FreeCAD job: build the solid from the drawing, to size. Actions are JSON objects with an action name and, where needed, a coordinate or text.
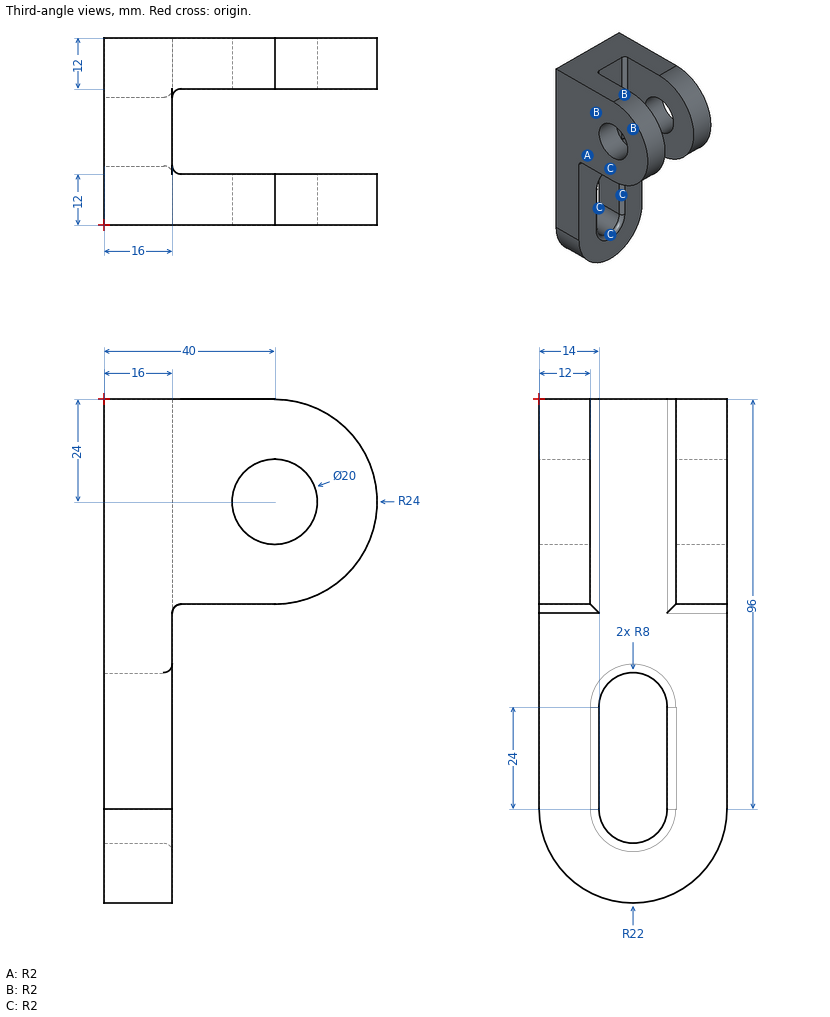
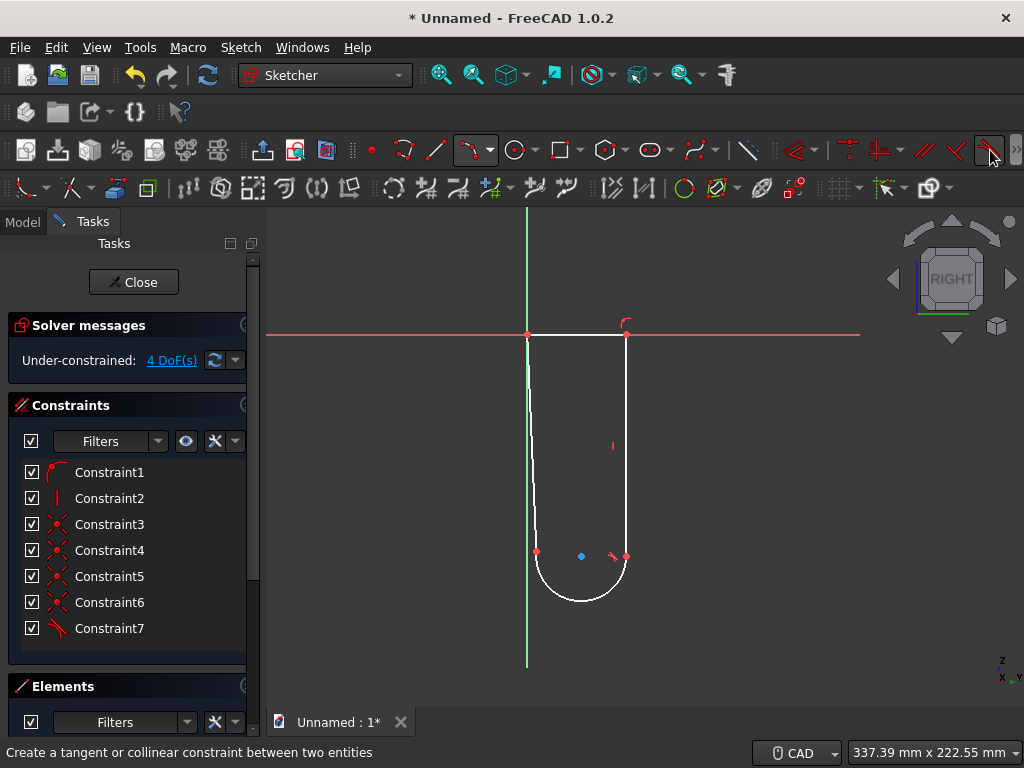
{"action": "left_click", "coordinate": [530, 400]}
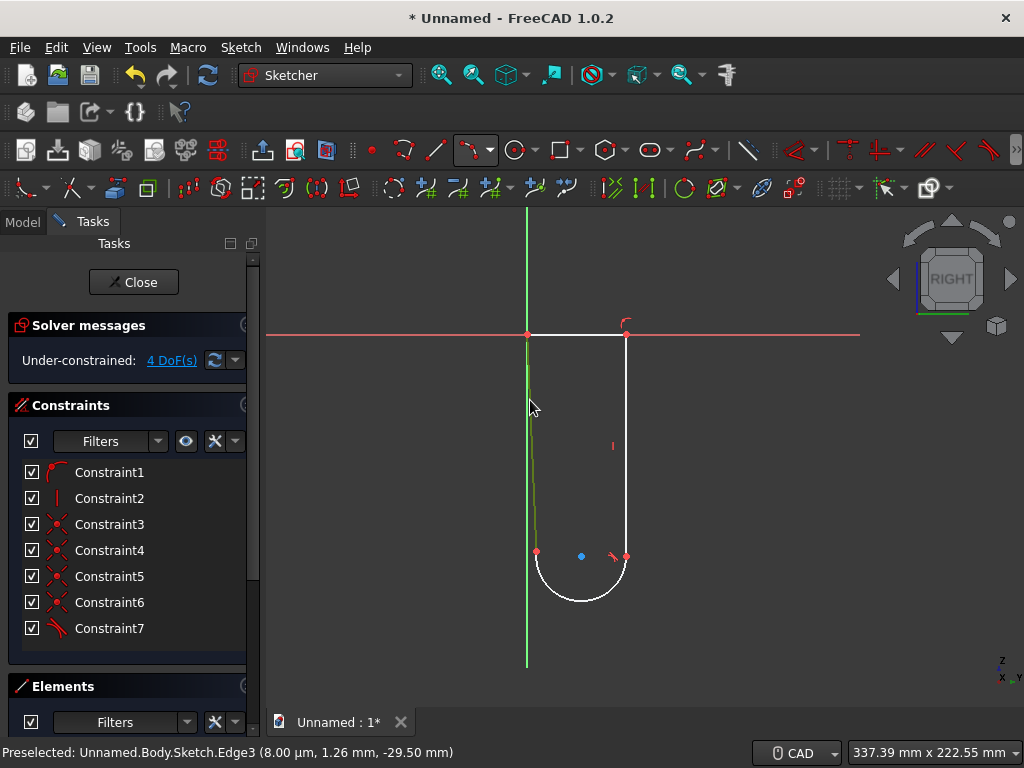
{"action": "left_click", "coordinate": [552, 591]}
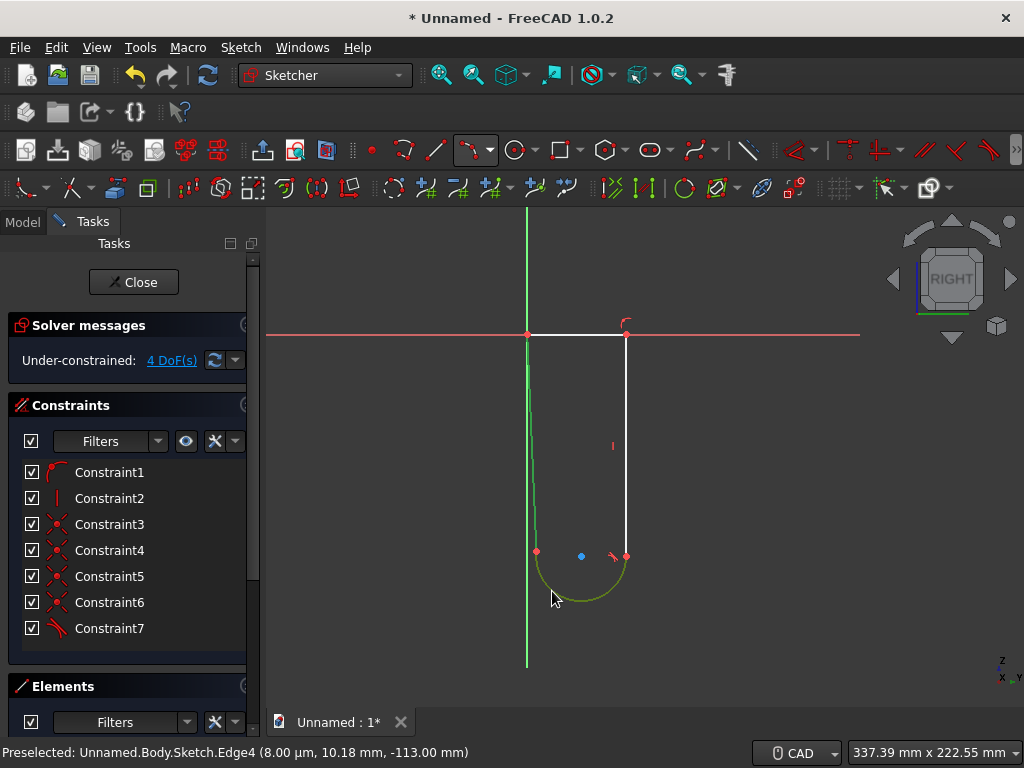
{"action": "left_click", "coordinate": [990, 150]}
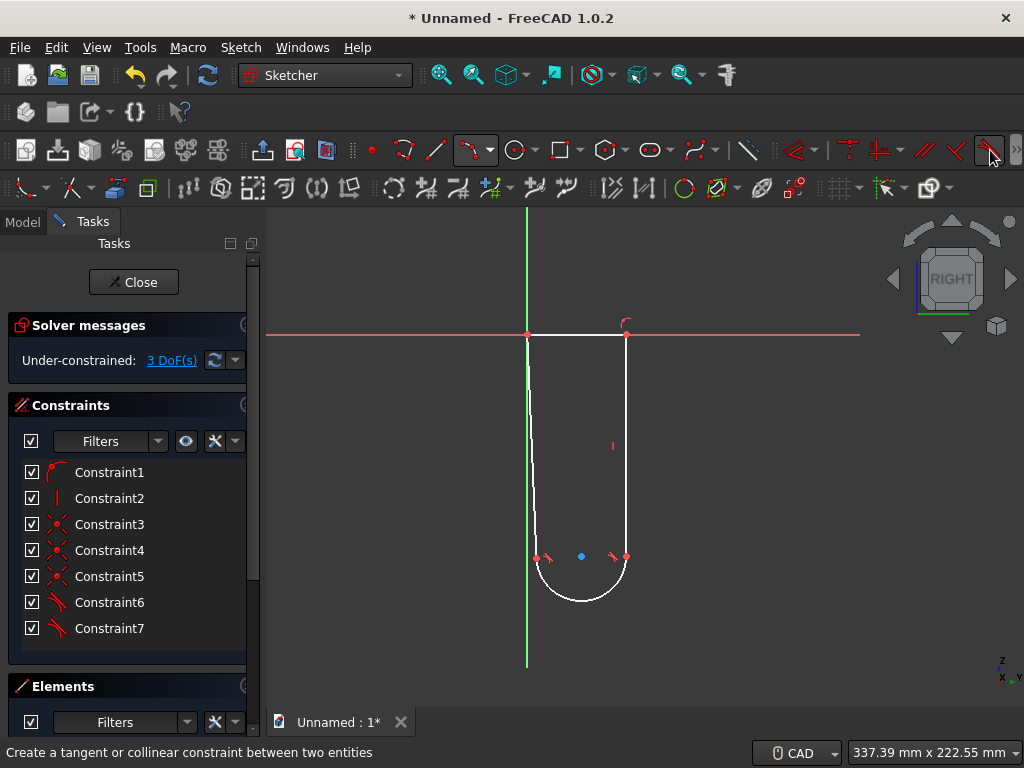
{"action": "left_click", "coordinate": [530, 402]}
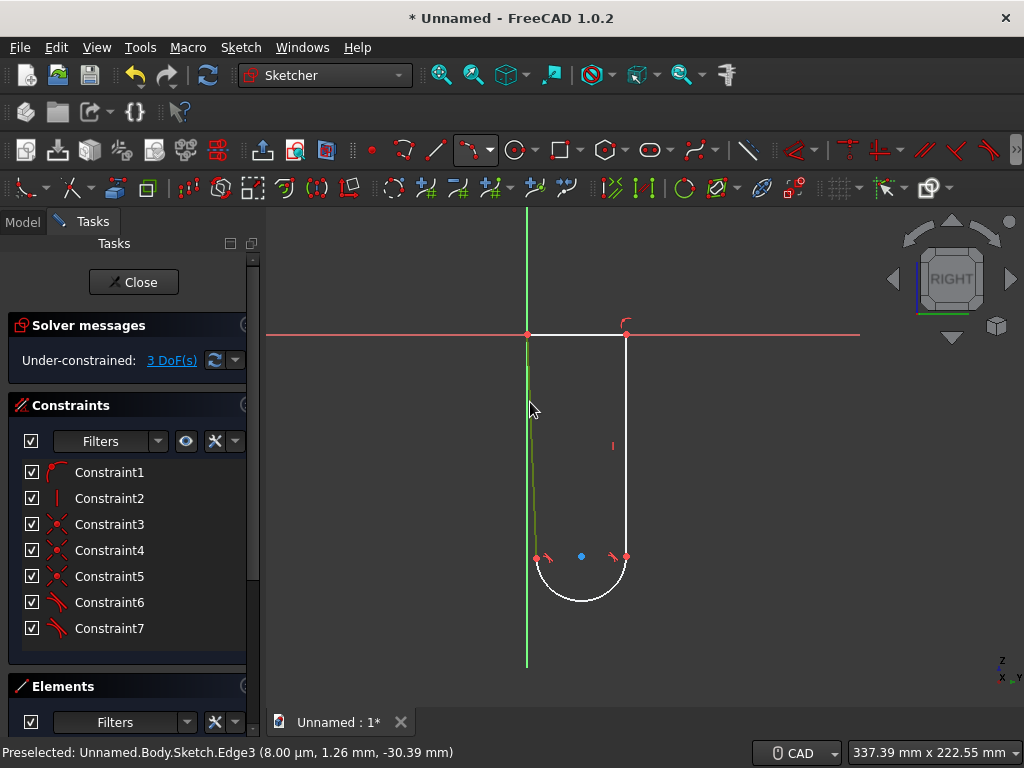
{"action": "left_click", "coordinate": [902, 150]}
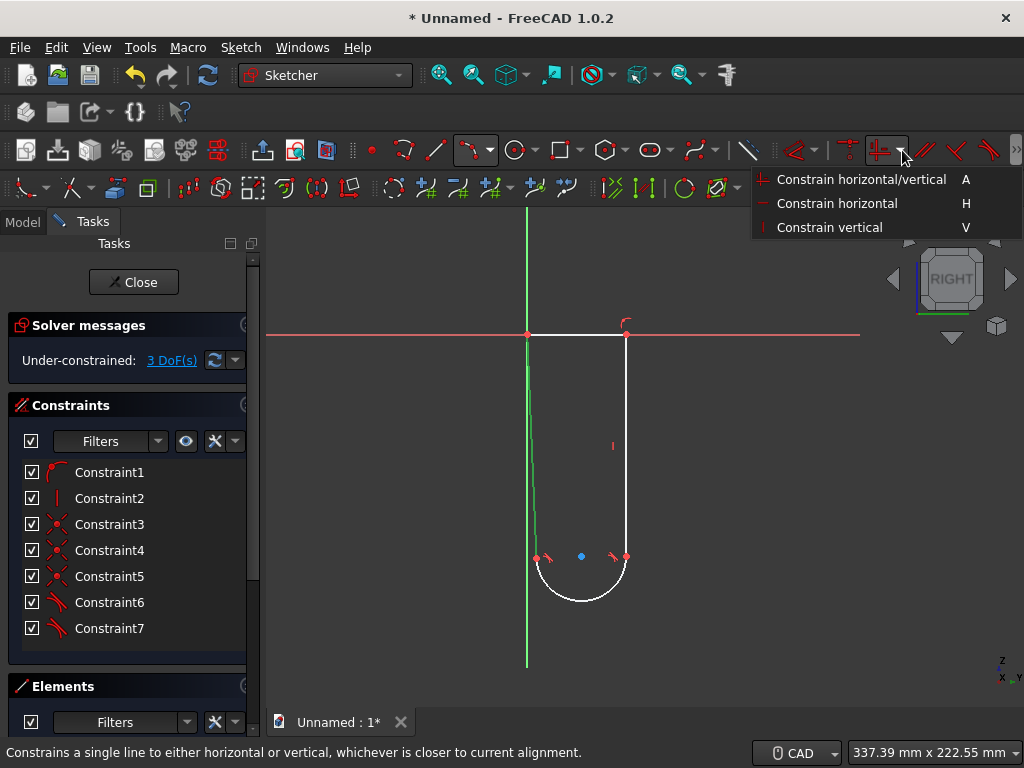
{"action": "left_click", "coordinate": [887, 227]}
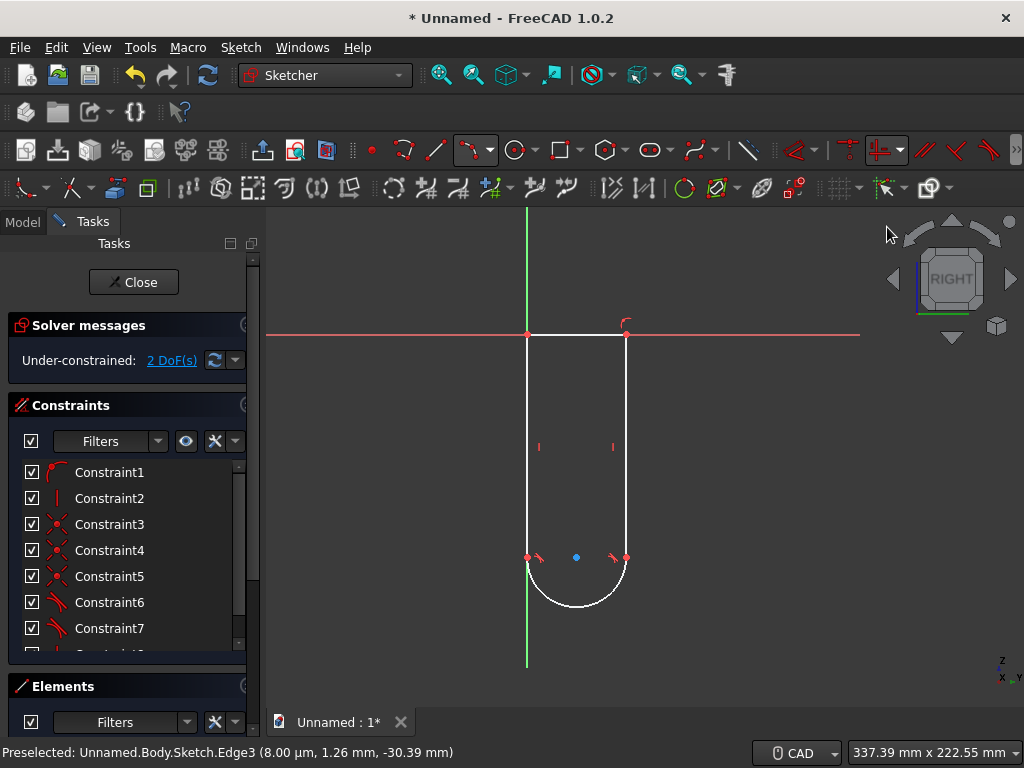
{"action": "left_click", "coordinate": [794, 150]}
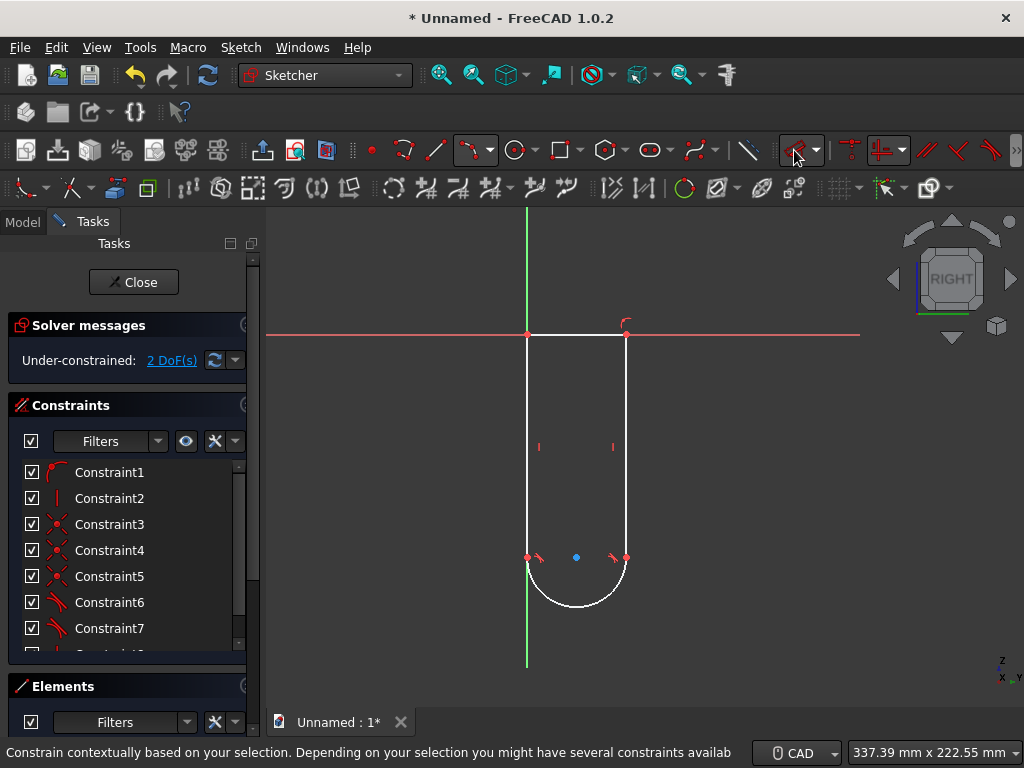
{"action": "left_click", "coordinate": [548, 598]}
{"action": "left_click", "coordinate": [503, 593]}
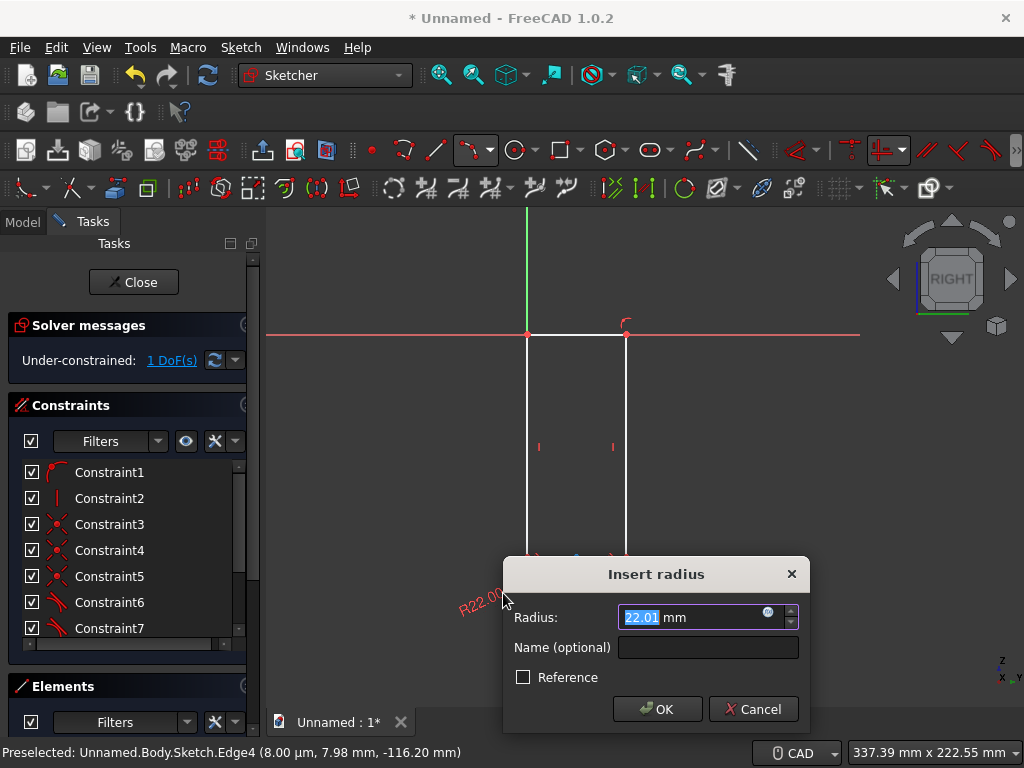
{"action": "type", "text": "22"}
{"action": "key", "text": "Return"}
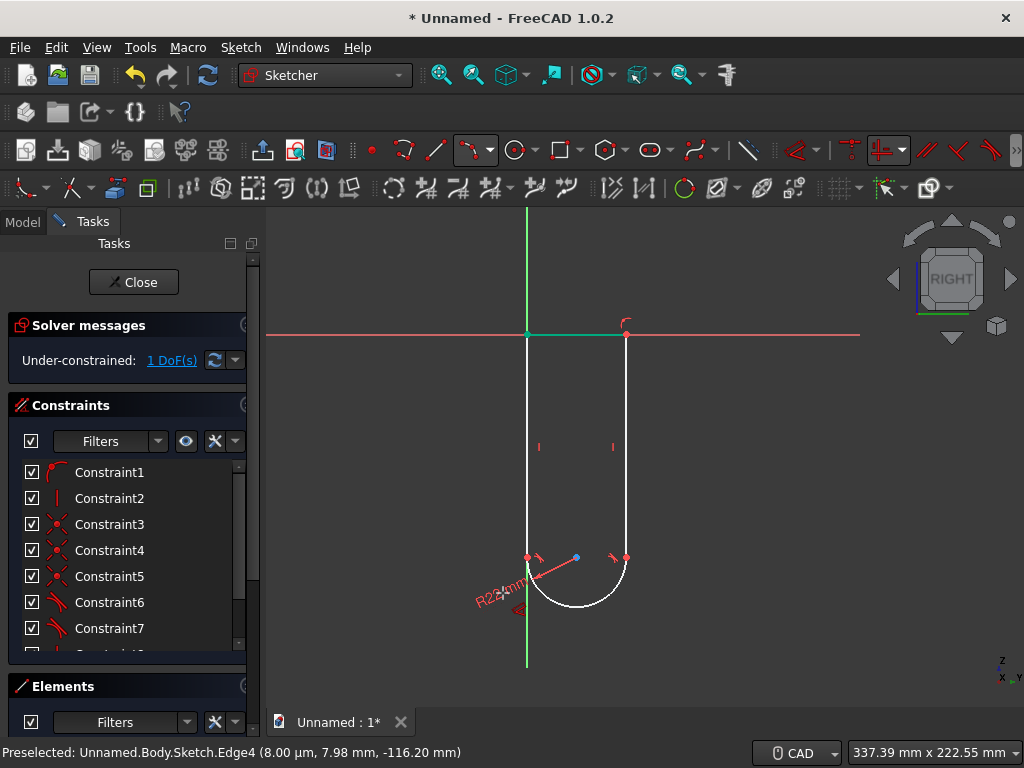
{"action": "left_click", "coordinate": [626, 491]}
{"action": "left_click", "coordinate": [660, 446]}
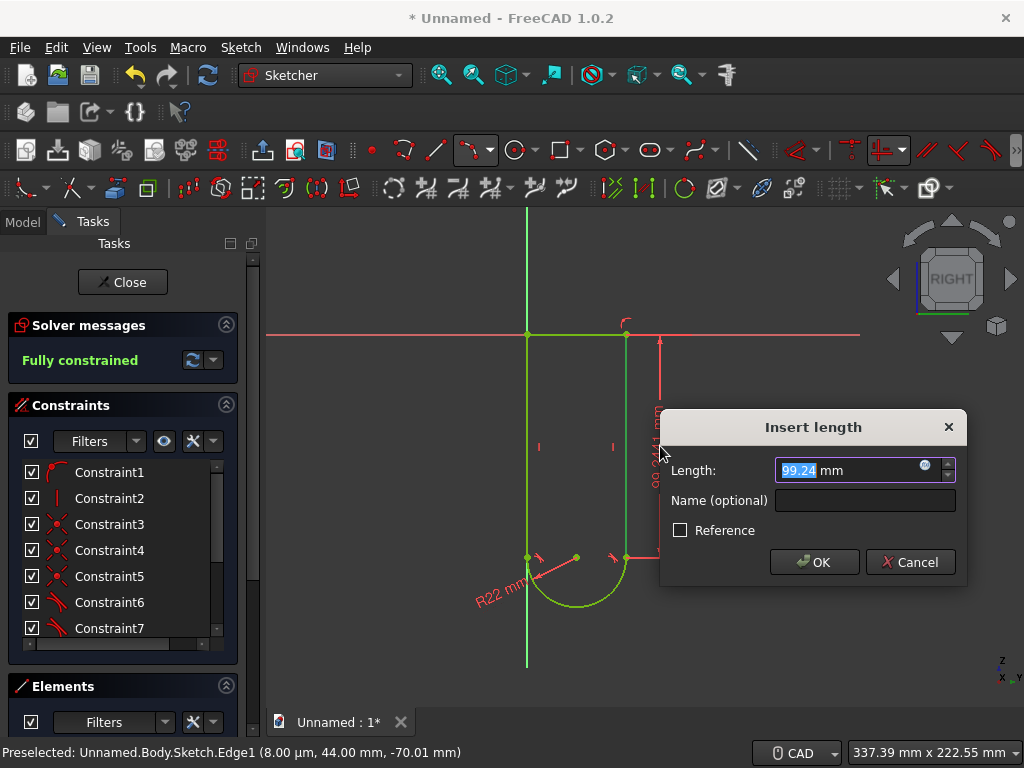
{"action": "type", "text": "96"}
{"action": "key", "text": "Return"}
{"action": "key", "text": "Escape"}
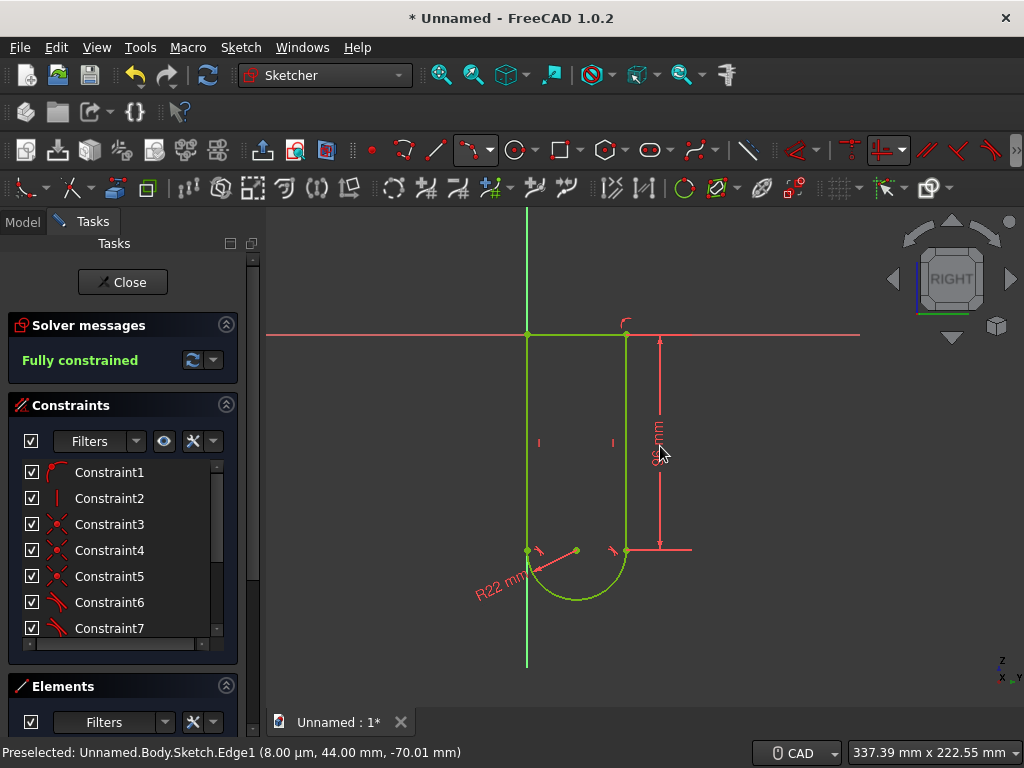
{"action": "left_click", "coordinate": [123, 282]}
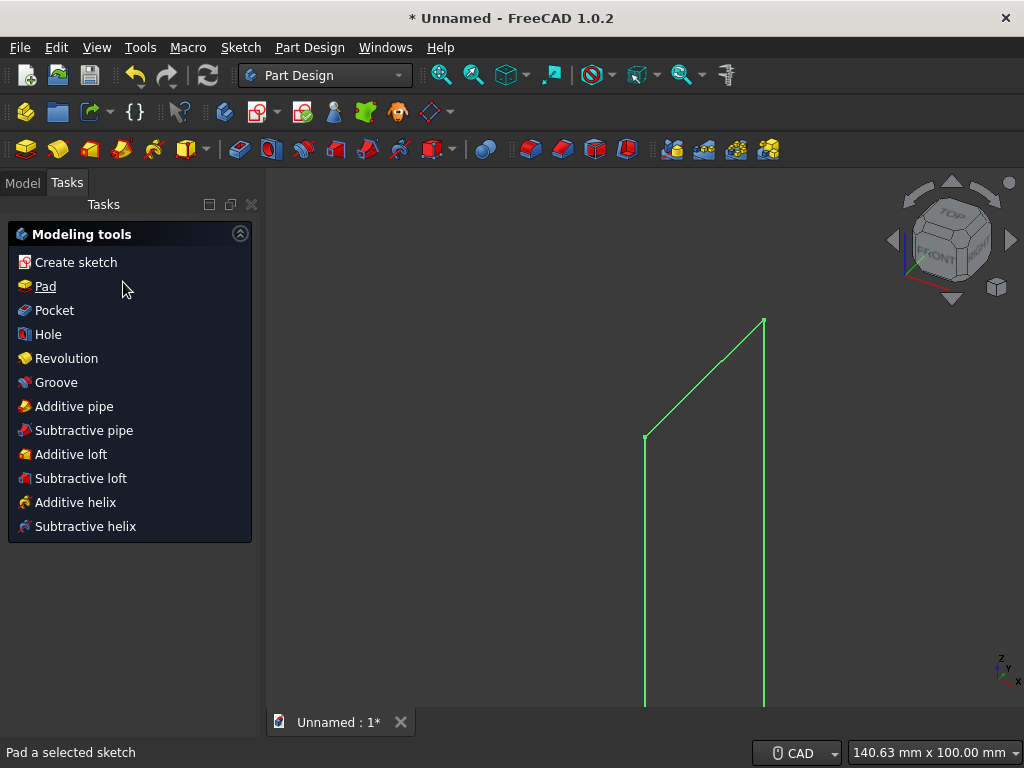
{"action": "left_click", "coordinate": [26, 150]}